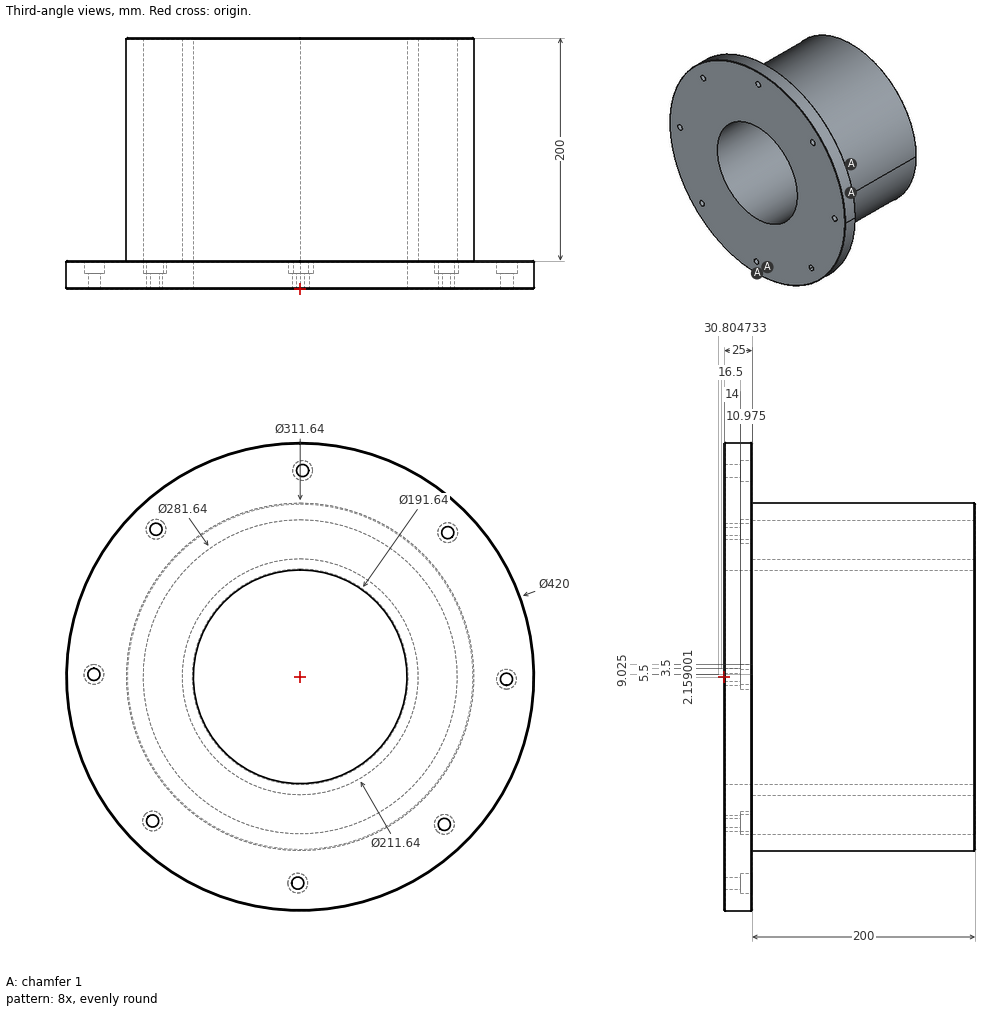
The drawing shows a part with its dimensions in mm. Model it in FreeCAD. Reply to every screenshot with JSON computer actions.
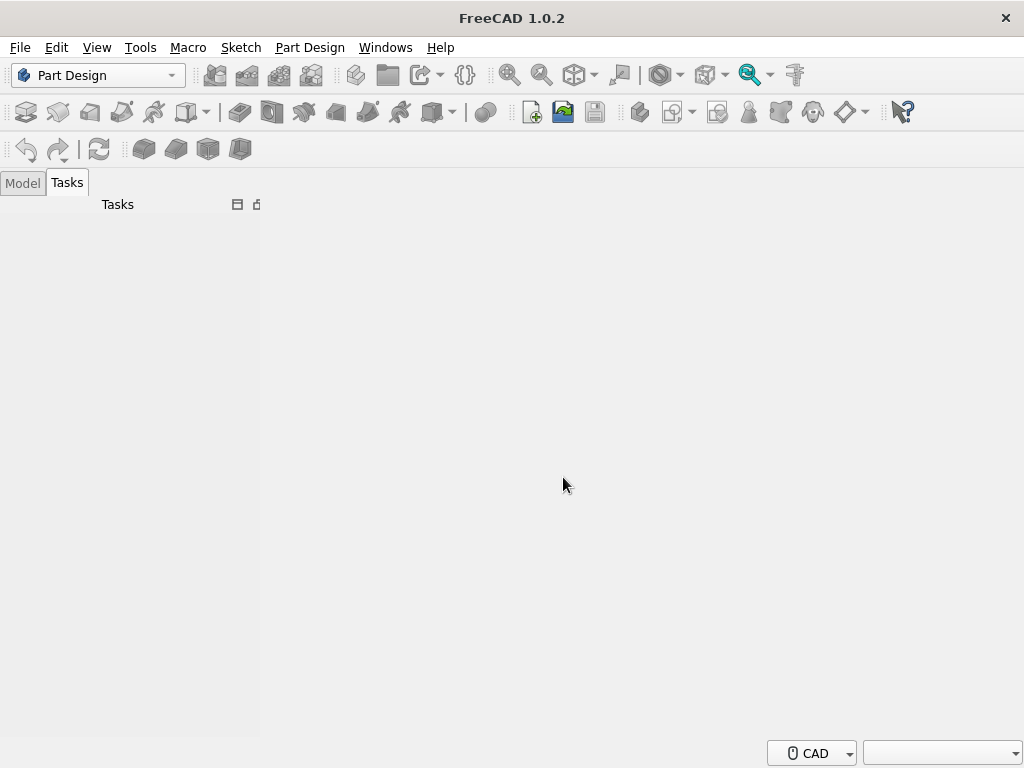
{"action": "left_click", "coordinate": [532, 112]}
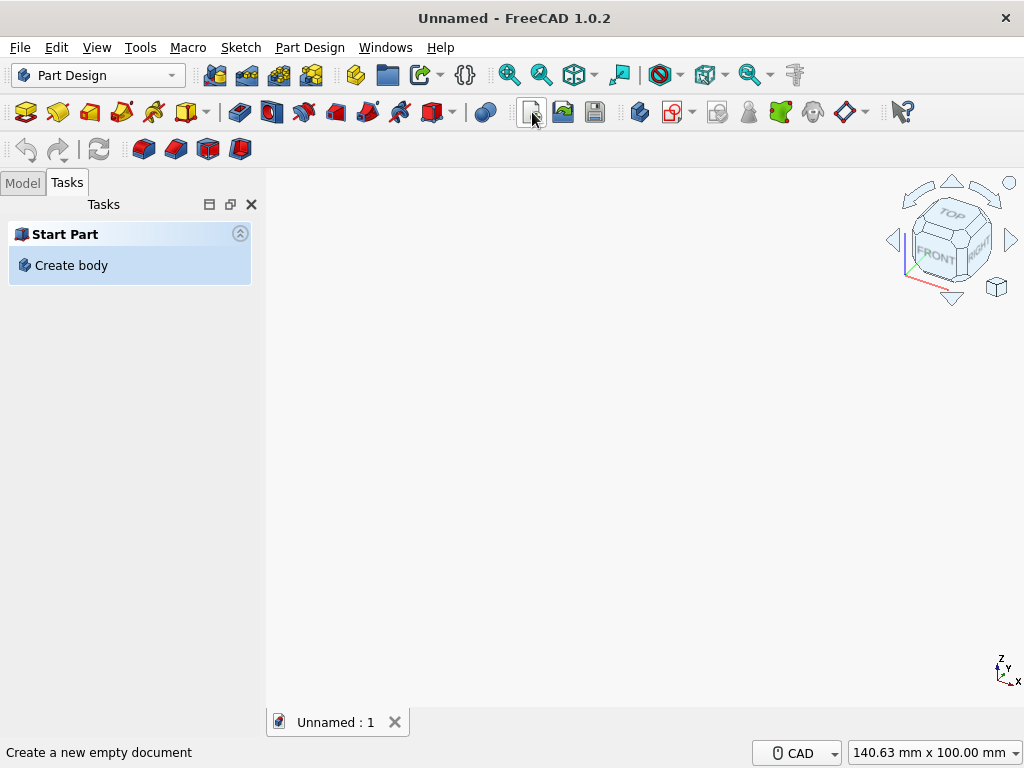
{"action": "left_click", "coordinate": [672, 112]}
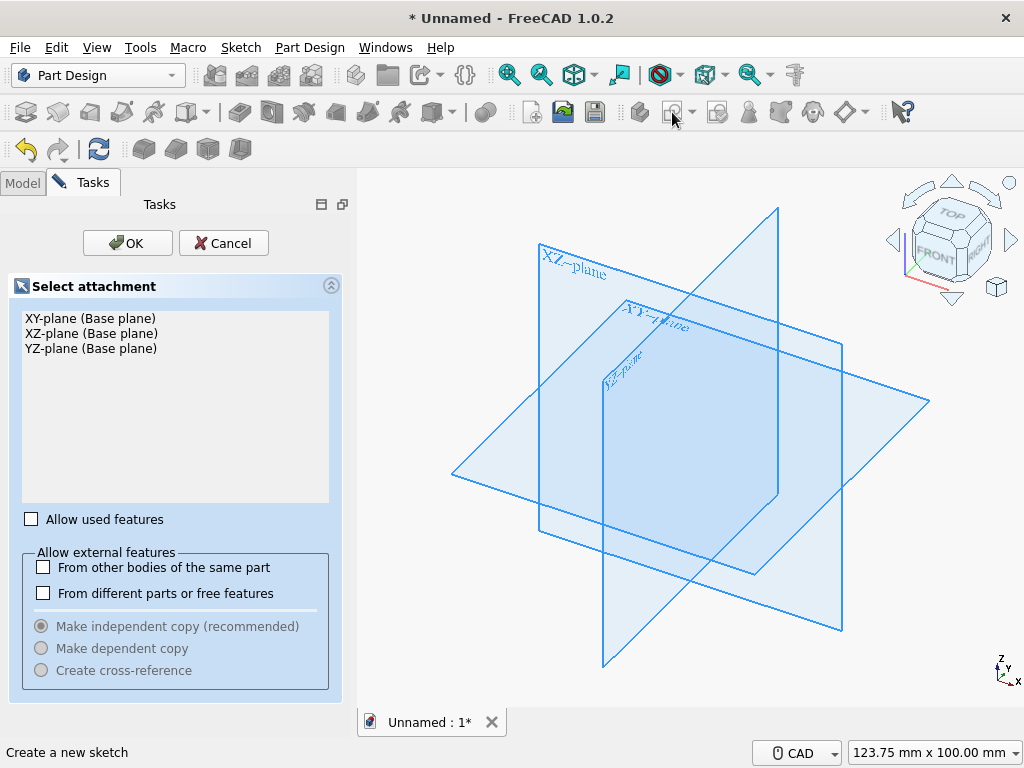
{"action": "left_click", "coordinate": [82, 334]}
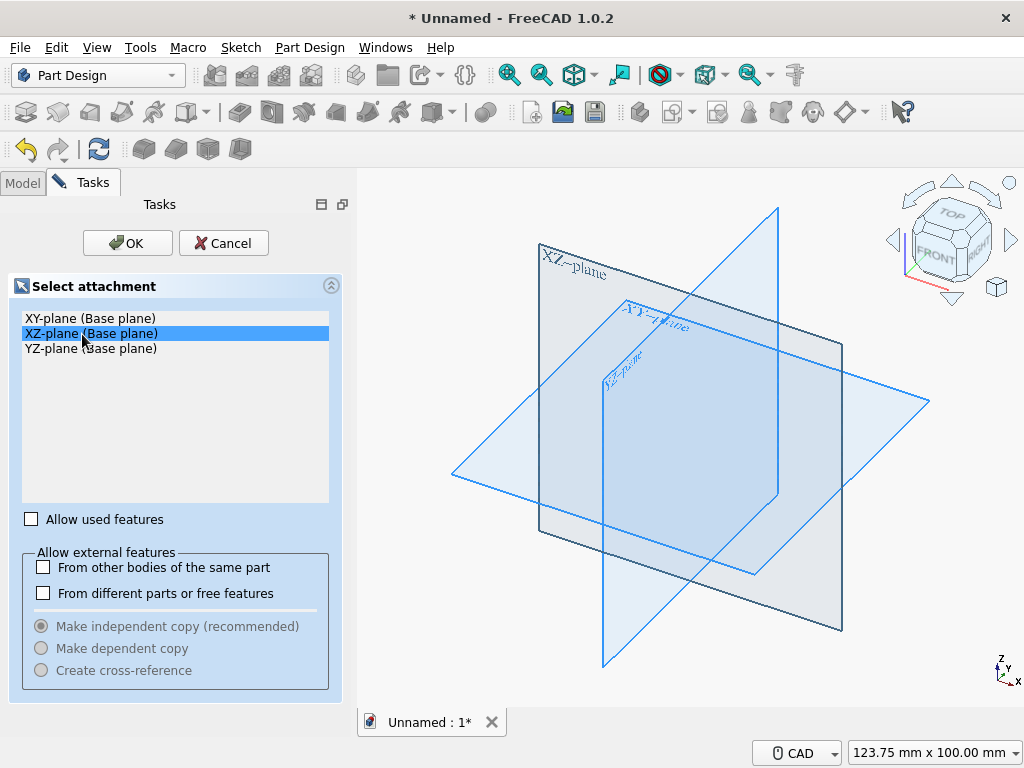
{"action": "left_click", "coordinate": [128, 243]}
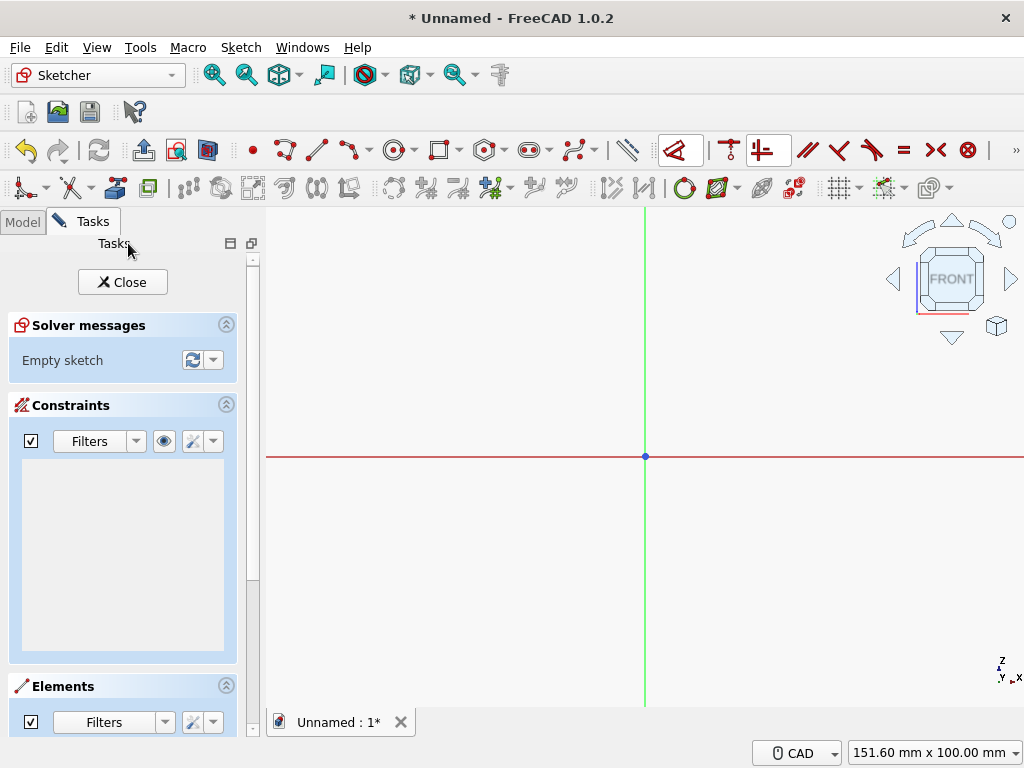
{"action": "scroll", "coordinate": [566, 457], "scroll_direction": "down", "scroll_amount": 10}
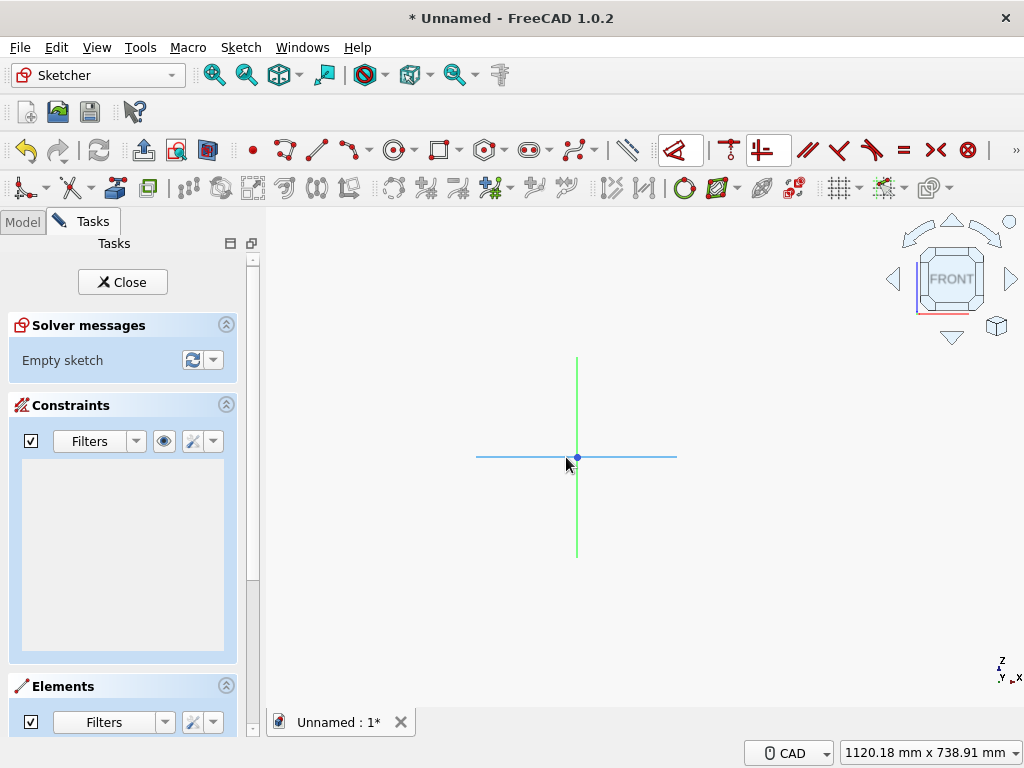
{"action": "left_click", "coordinate": [394, 150]}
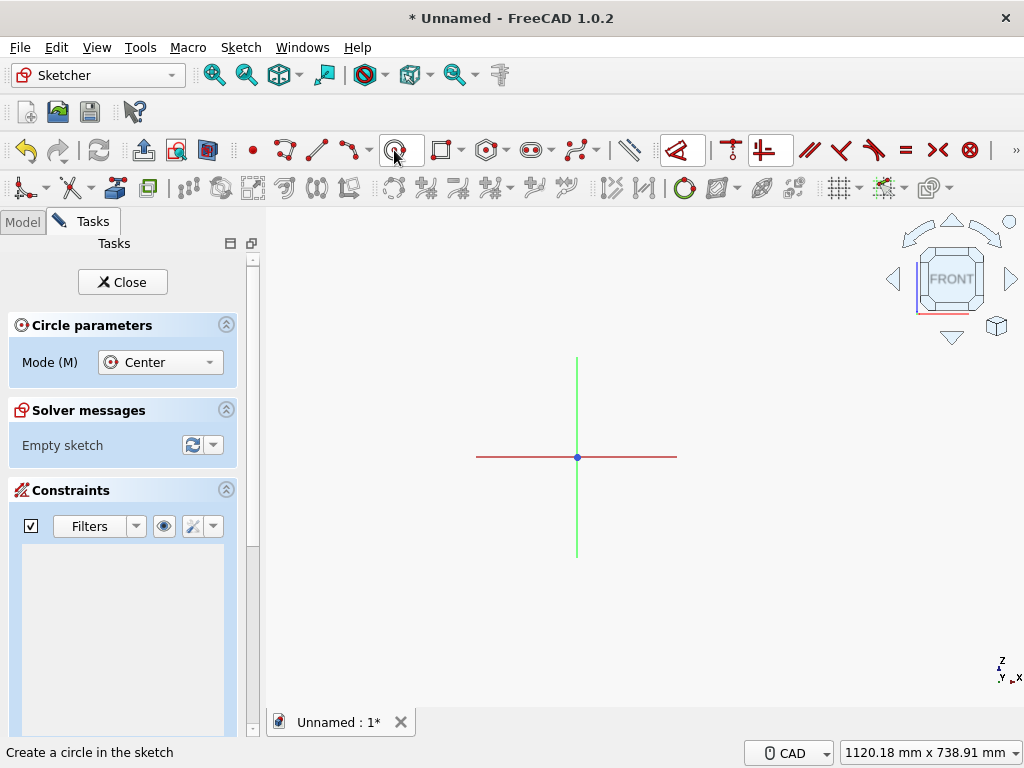
{"action": "left_click", "coordinate": [577, 457]}
{"action": "left_click", "coordinate": [678, 357]}
{"action": "key", "text": "Escape"}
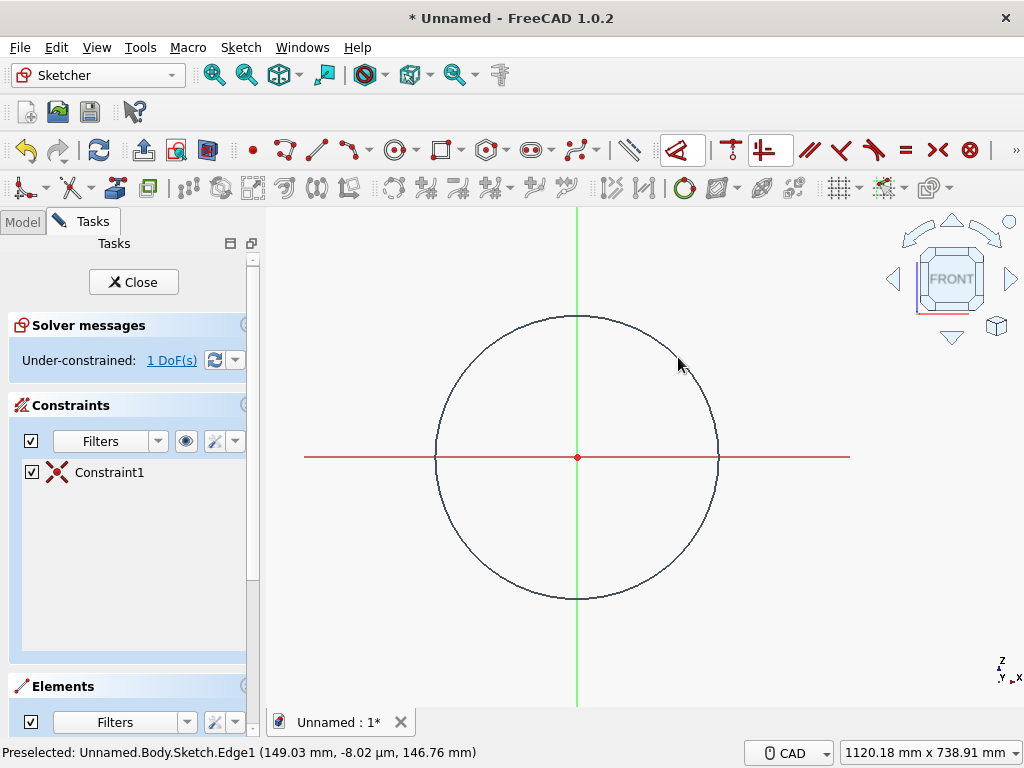
{"action": "left_click", "coordinate": [676, 150]}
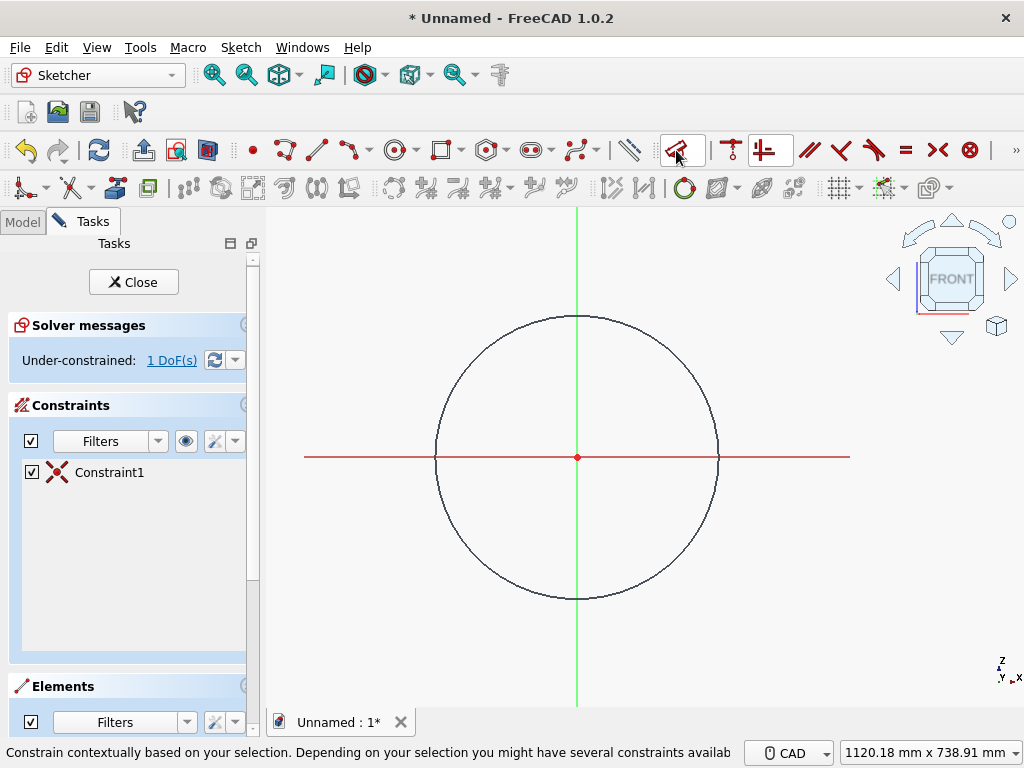
{"action": "left_click", "coordinate": [677, 357]}
{"action": "left_click", "coordinate": [700, 334]}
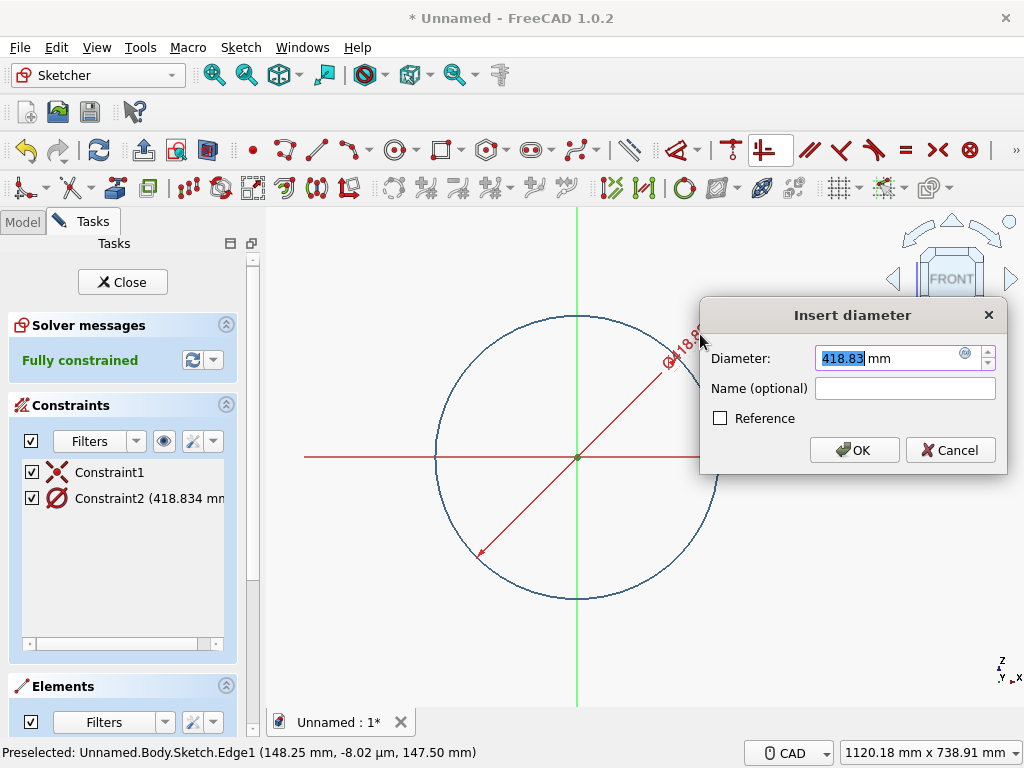
{"action": "type", "text": "420"}
{"action": "key", "text": "Return"}
{"action": "key", "text": "Escape"}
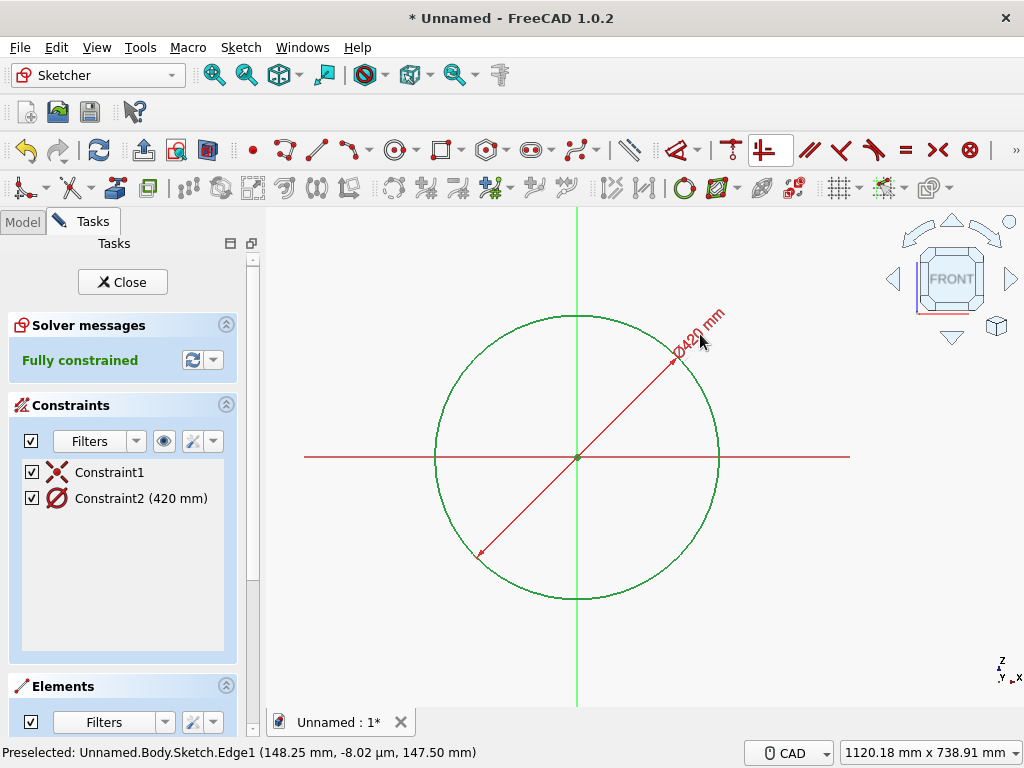
{"action": "left_click", "coordinate": [123, 282]}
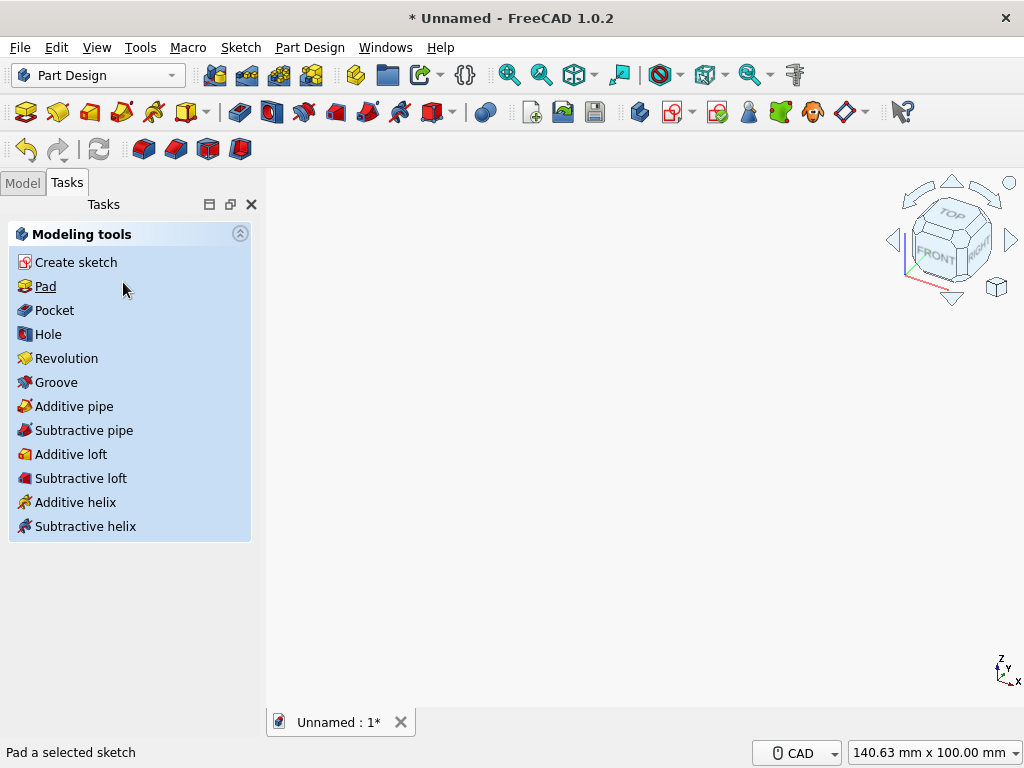
{"action": "left_click", "coordinate": [26, 112]}